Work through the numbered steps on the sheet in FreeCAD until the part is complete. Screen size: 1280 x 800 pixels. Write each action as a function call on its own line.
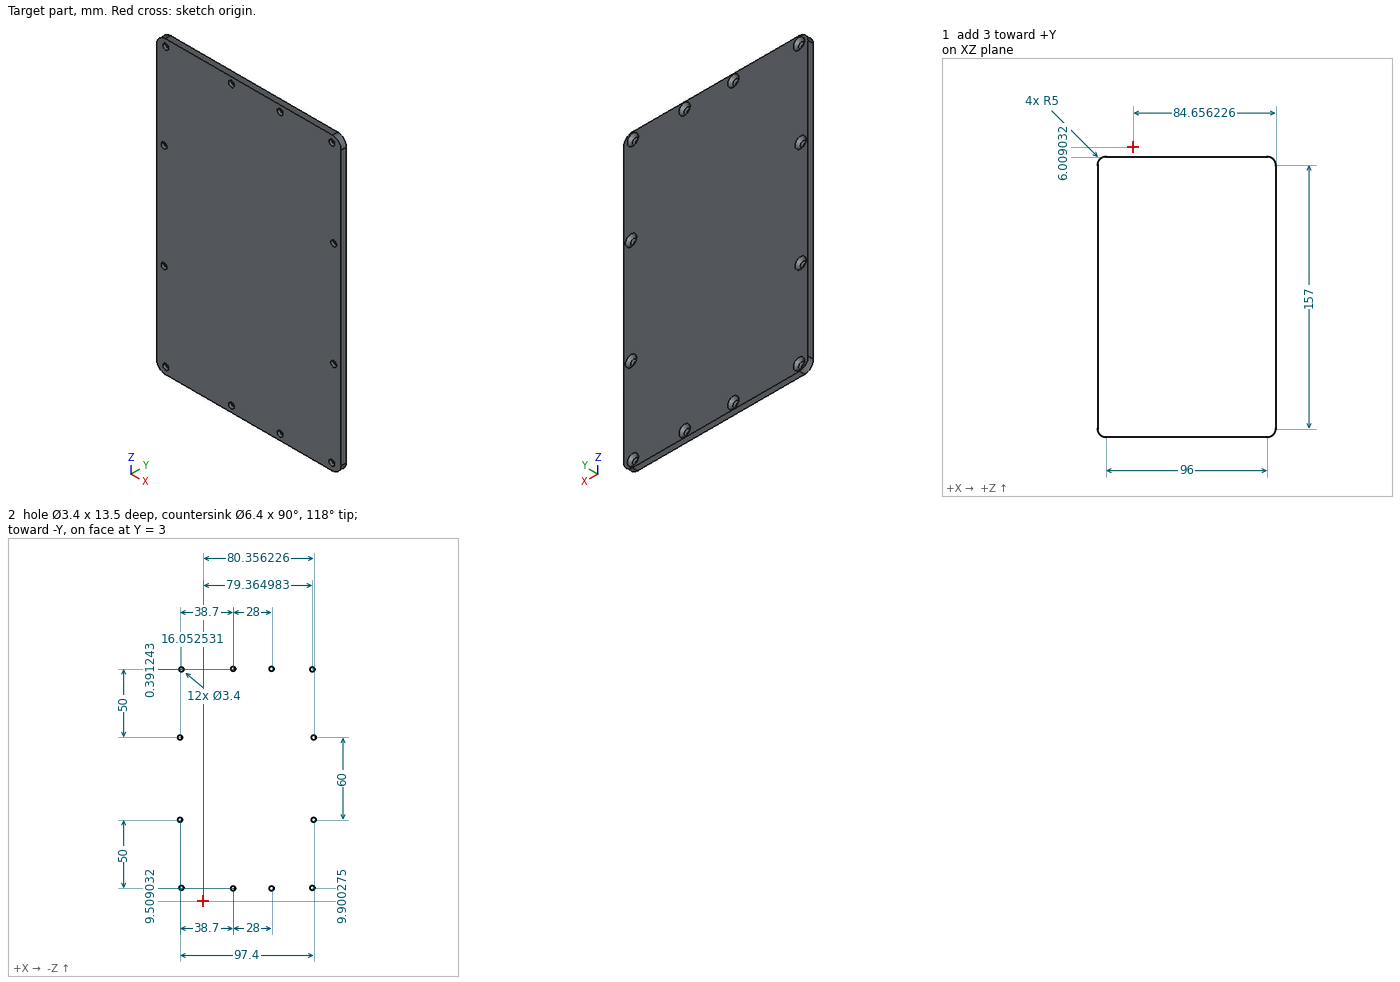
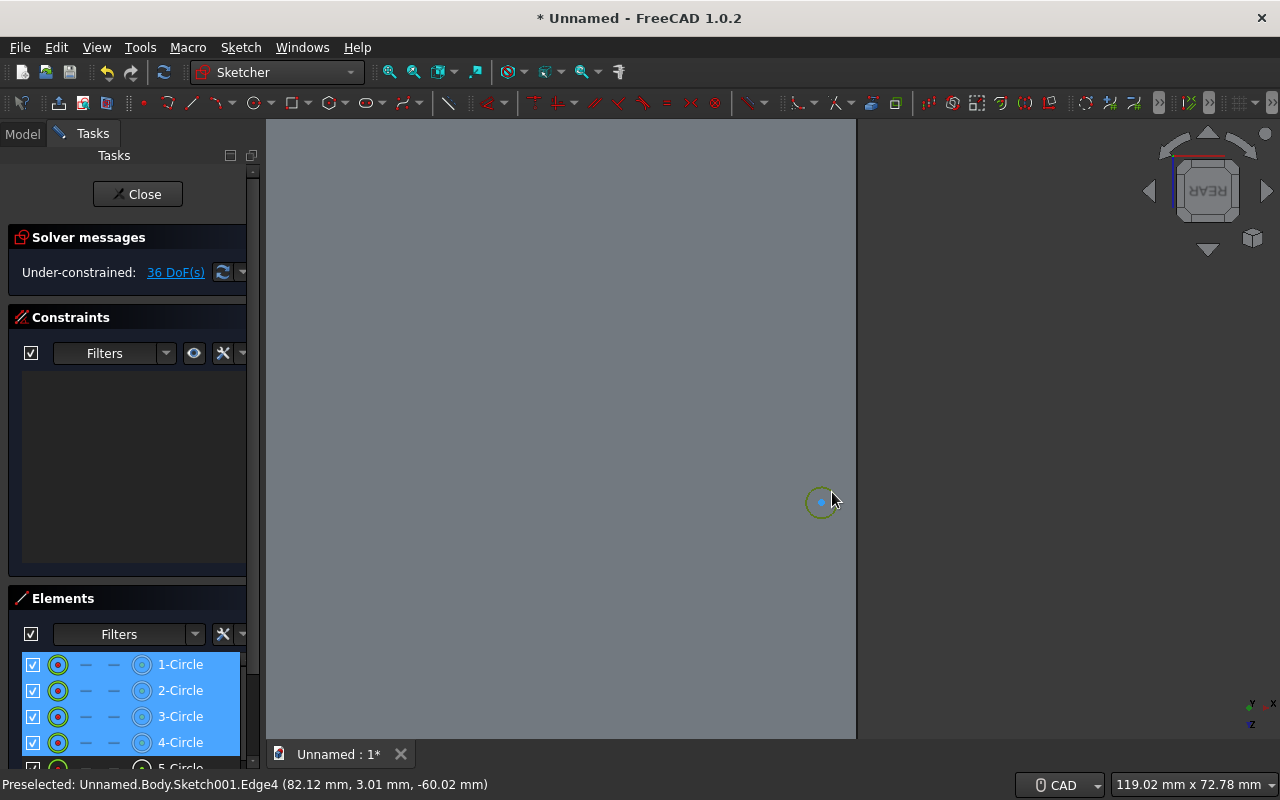
scroll(834, 494, down, 6)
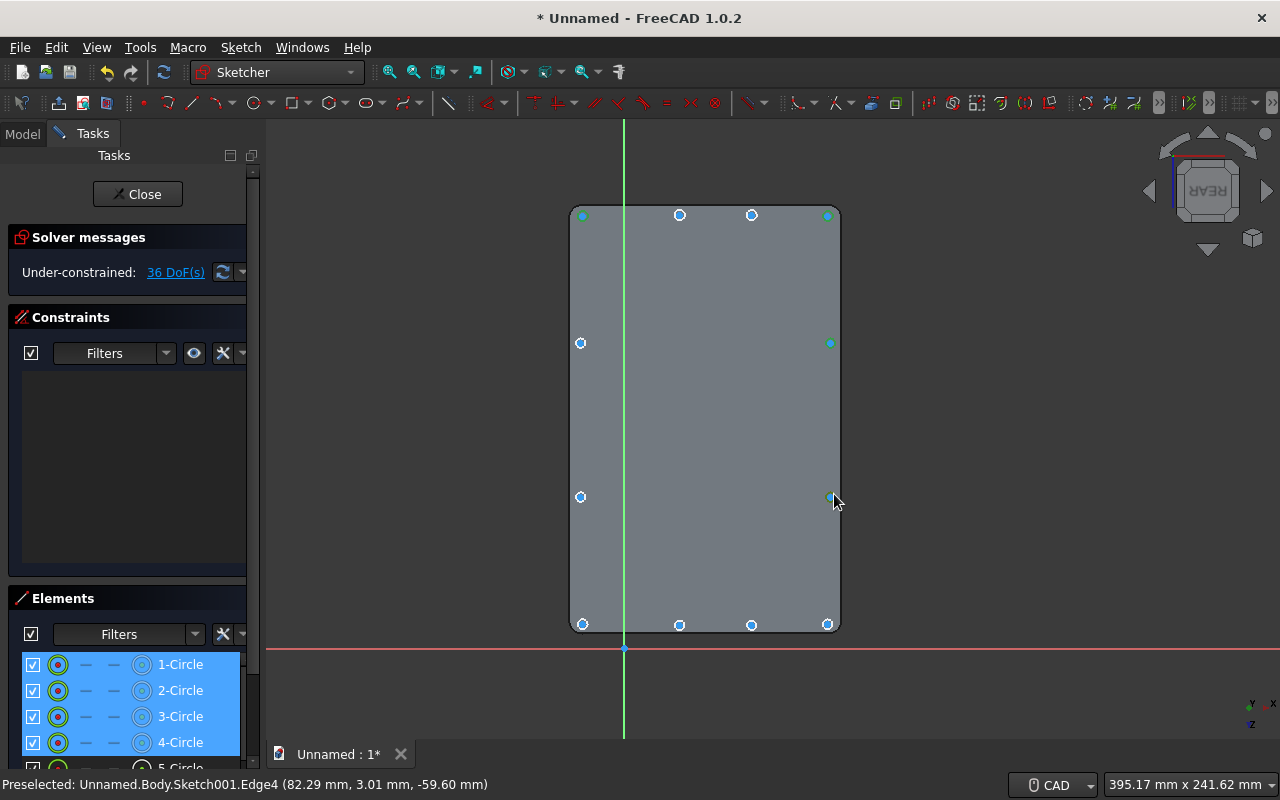
scroll(831, 621, up, 6)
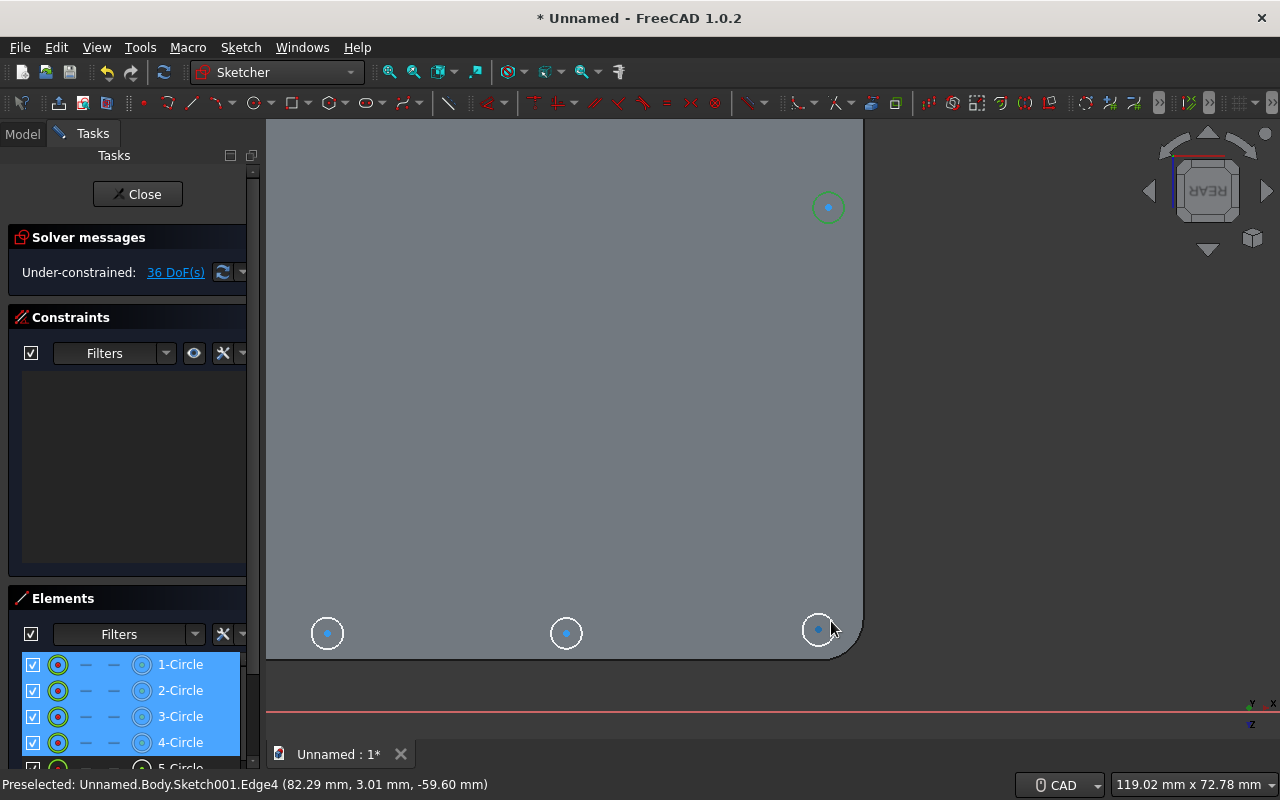
click(830, 619)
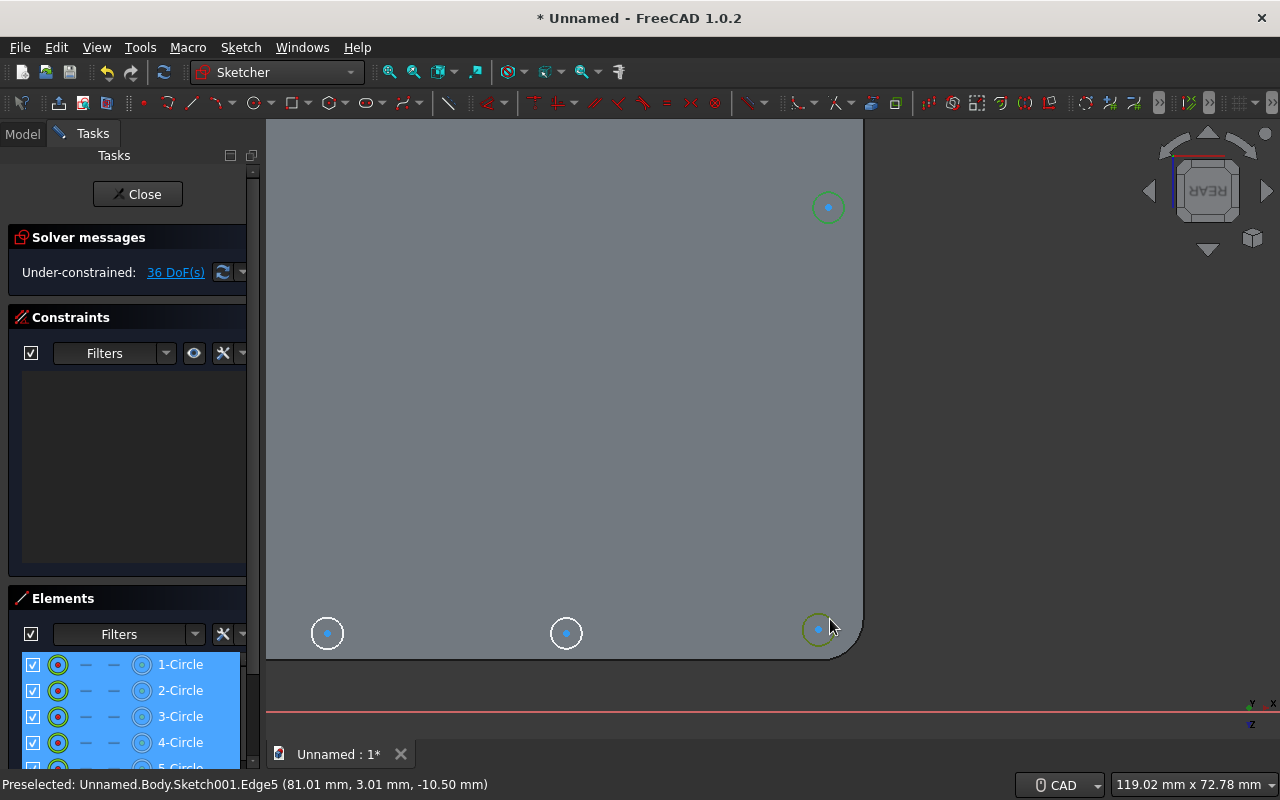
scroll(831, 621, down, 6)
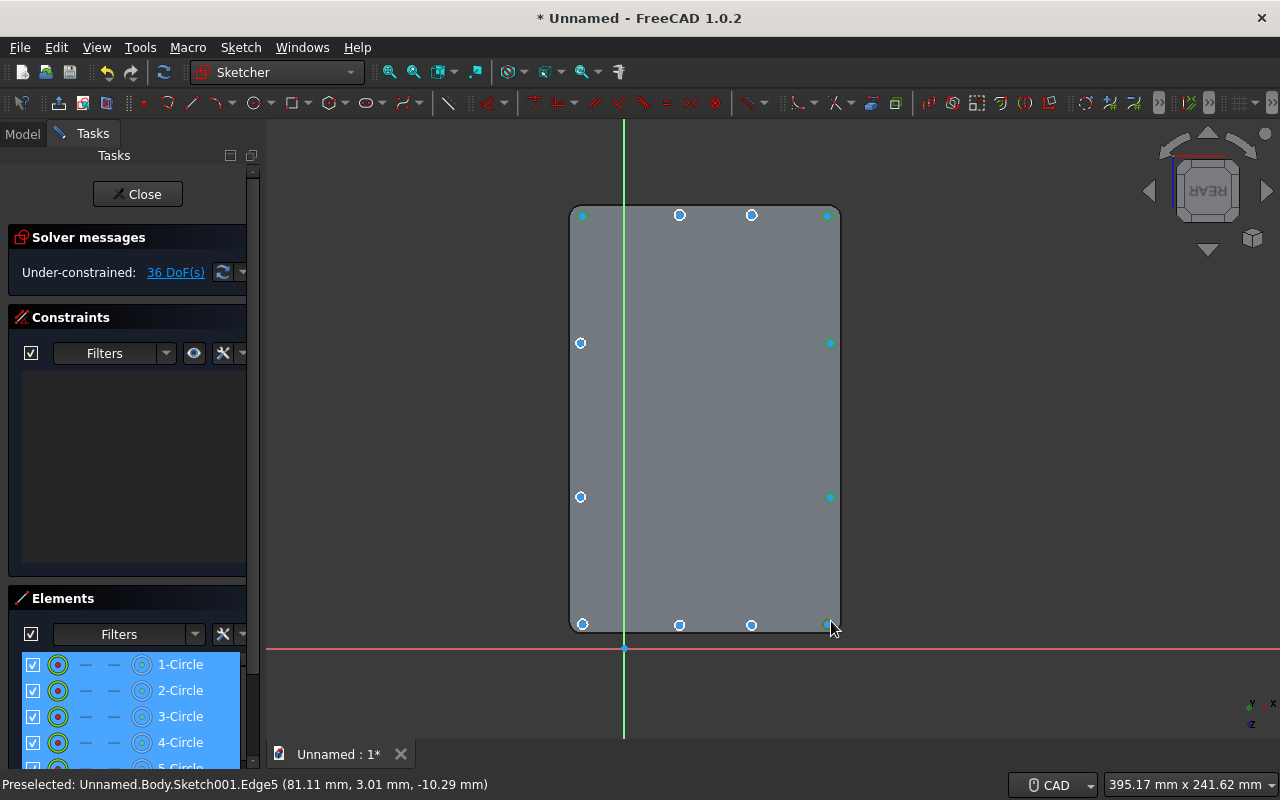
scroll(586, 621, up, 6)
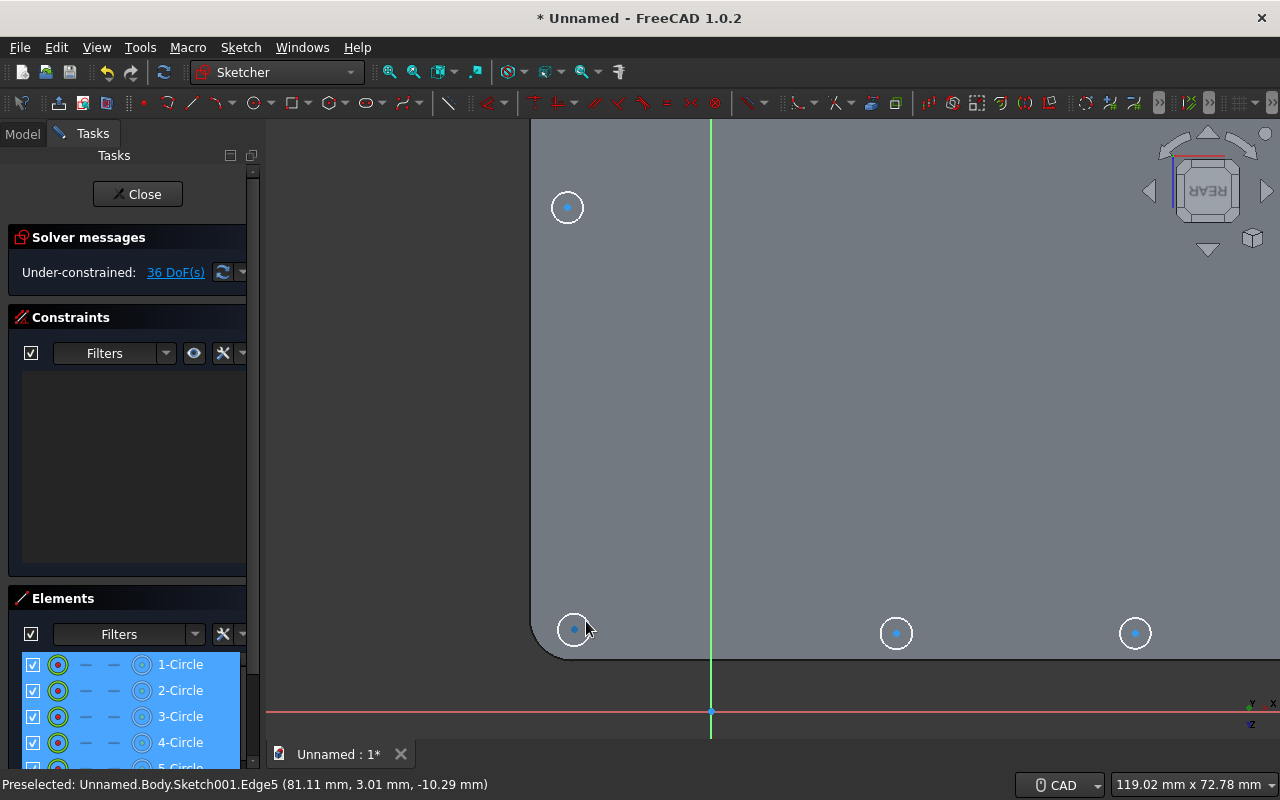
click(586, 618)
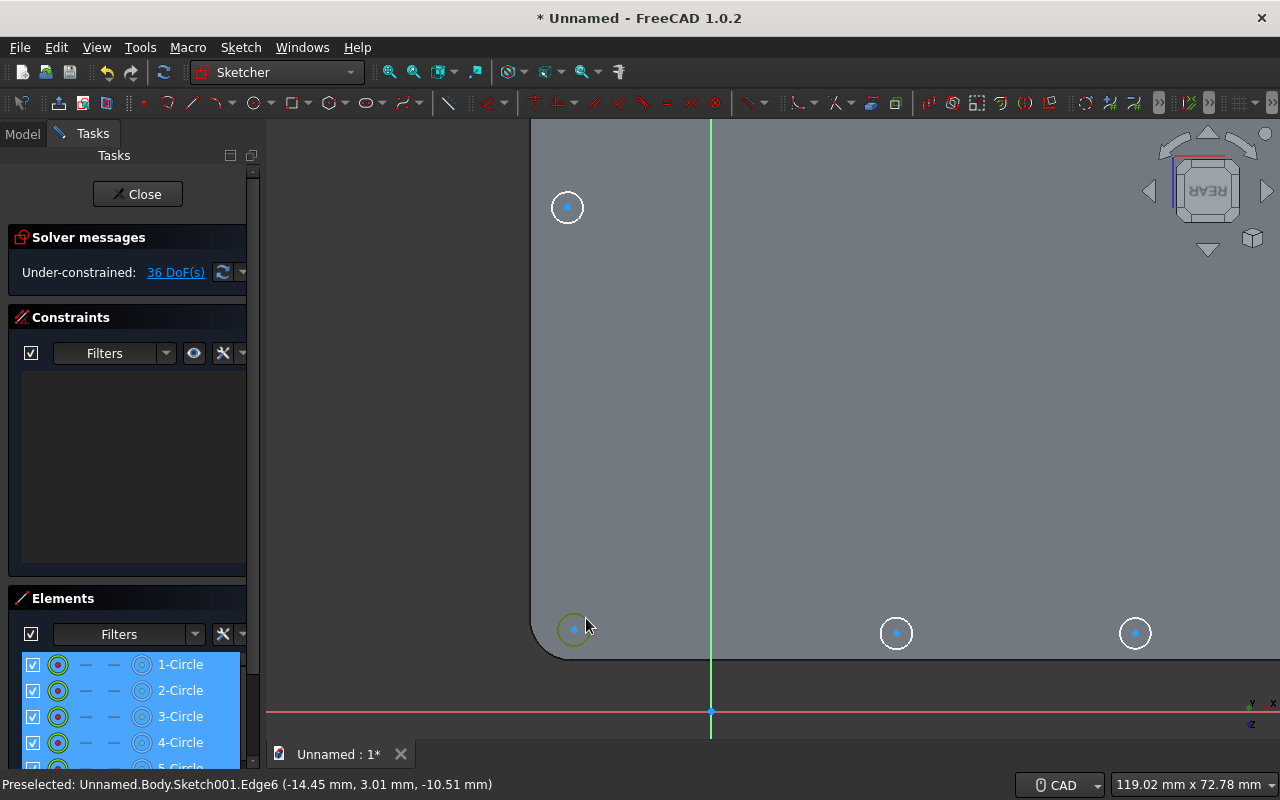
click(578, 197)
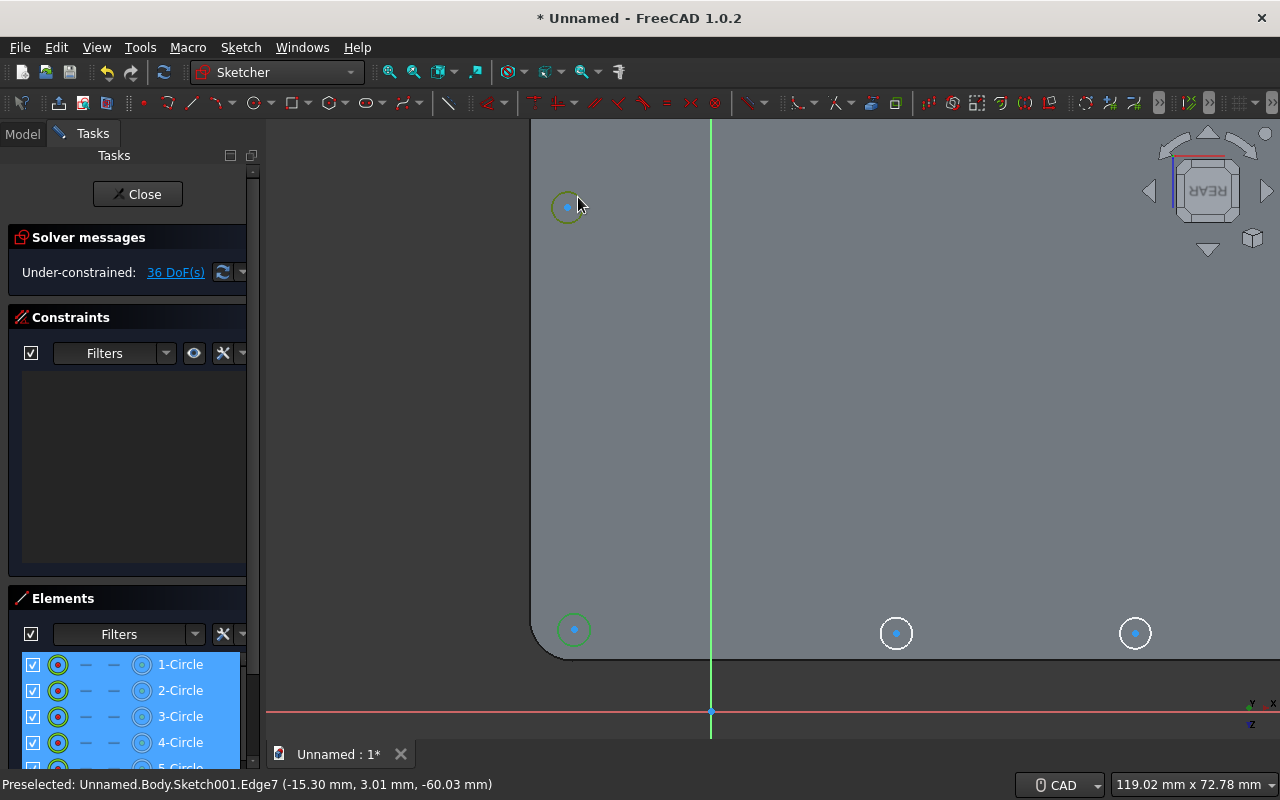
scroll(585, 621, down, 6)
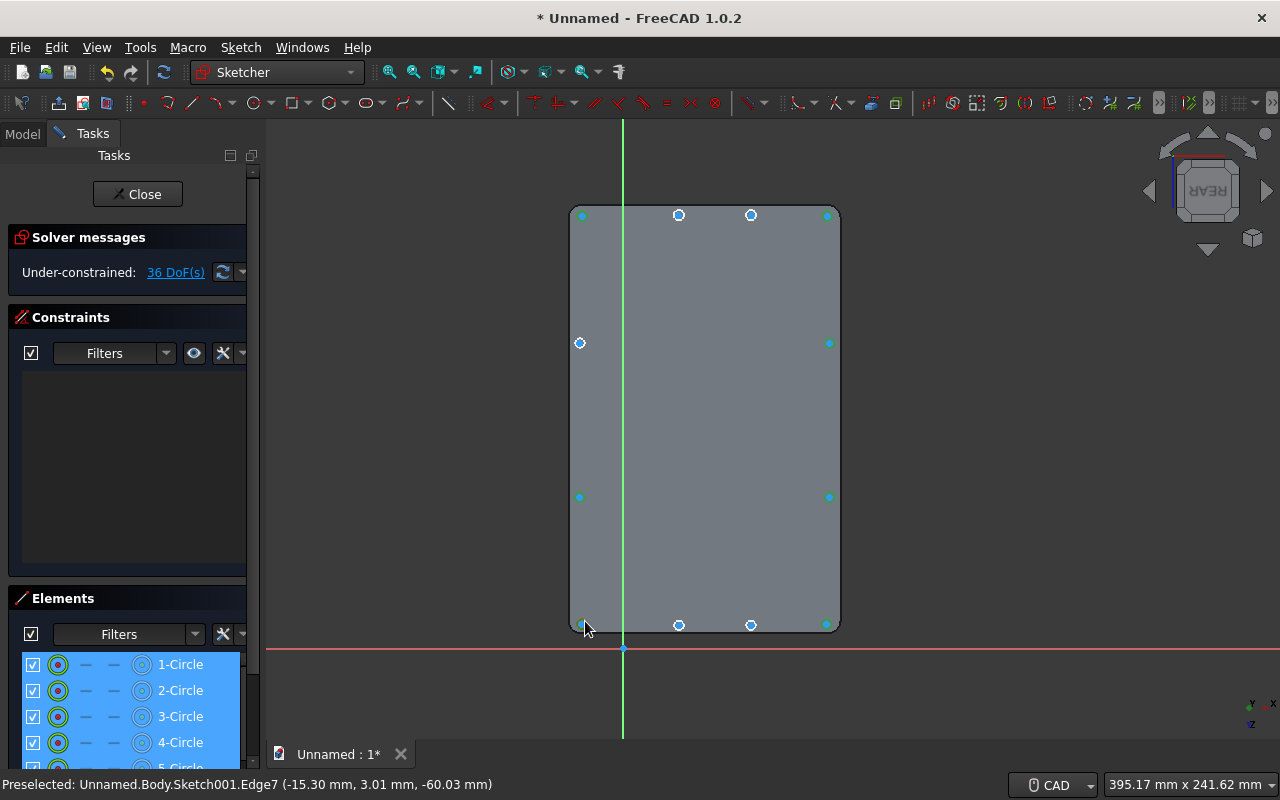
scroll(583, 340, up, 6)